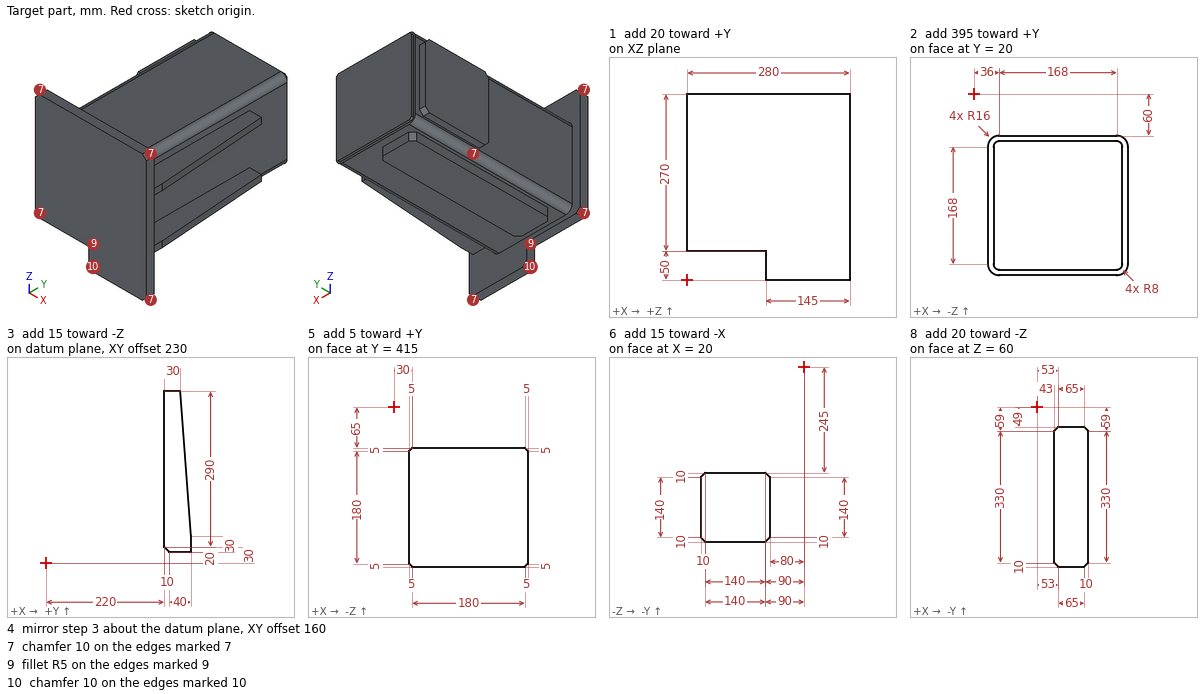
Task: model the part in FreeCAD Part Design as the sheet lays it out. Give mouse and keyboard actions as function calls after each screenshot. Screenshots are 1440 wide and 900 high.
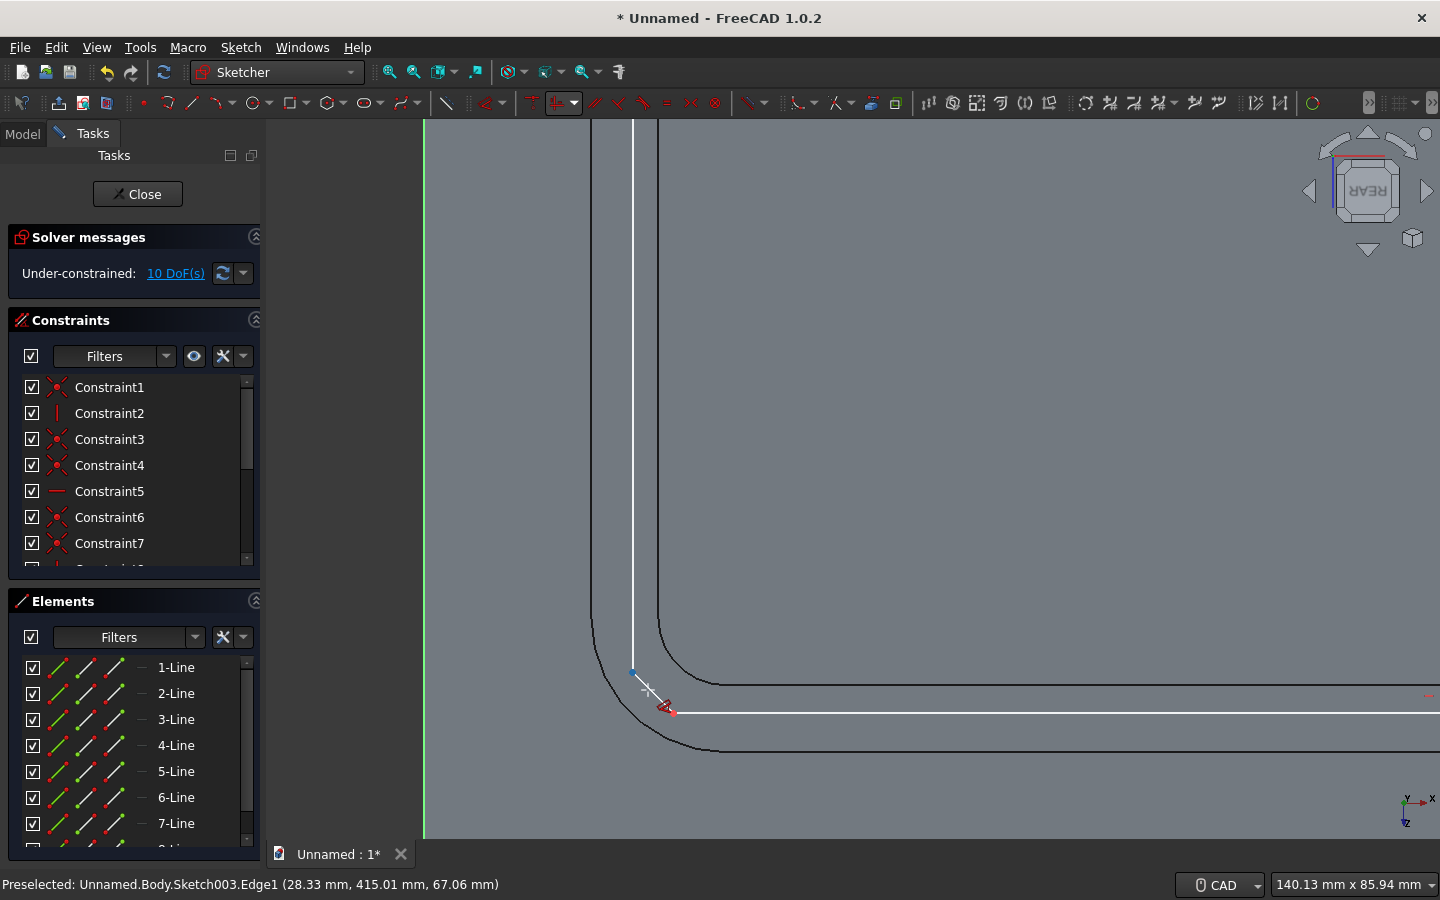
click(645, 685)
click(653, 747)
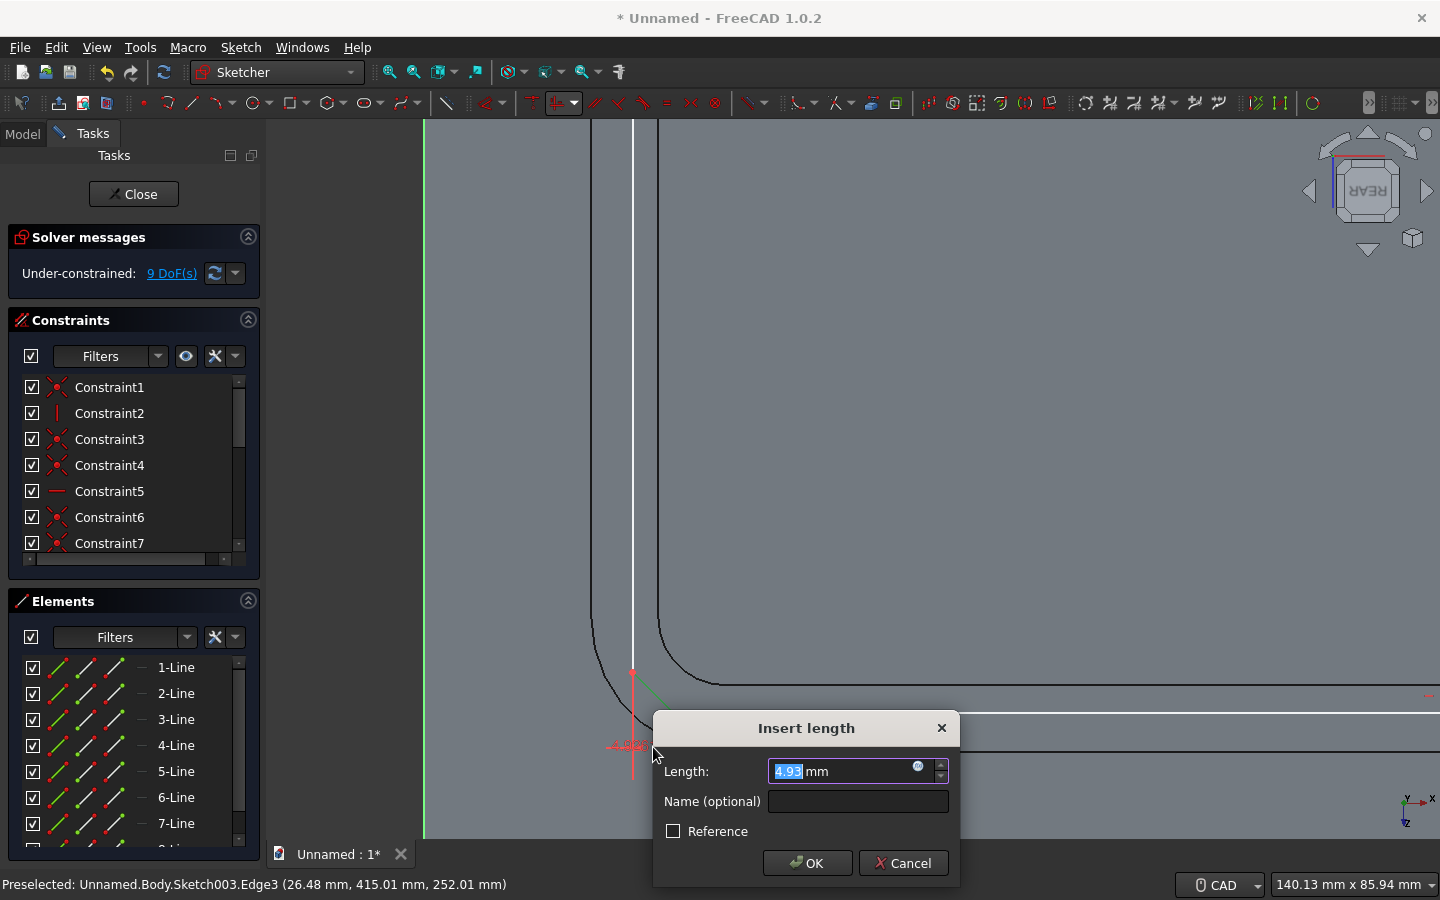
text(5)
key(Return)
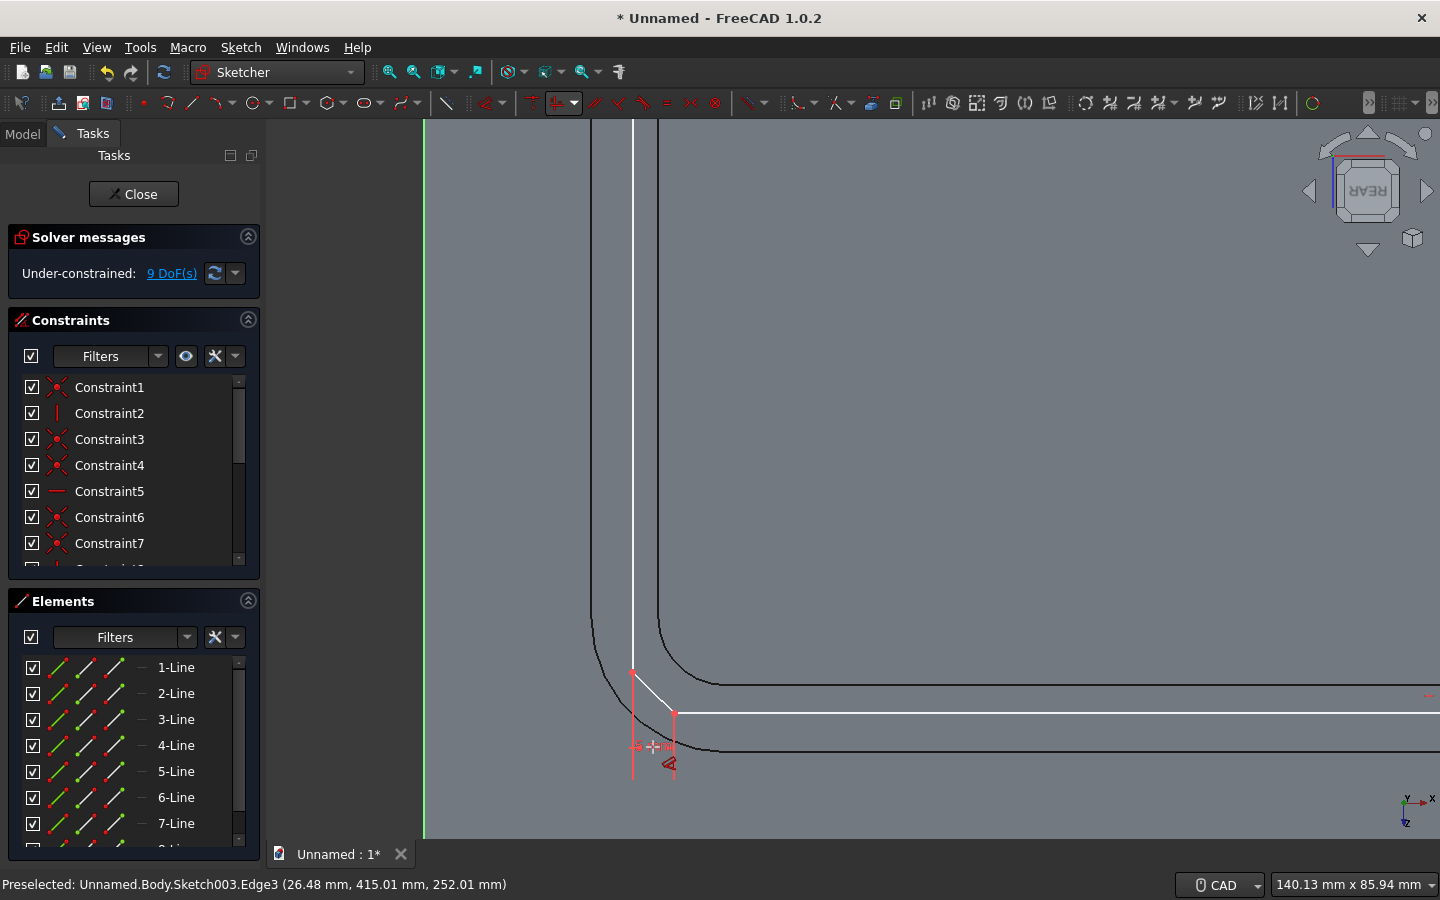
click(645, 685)
click(599, 693)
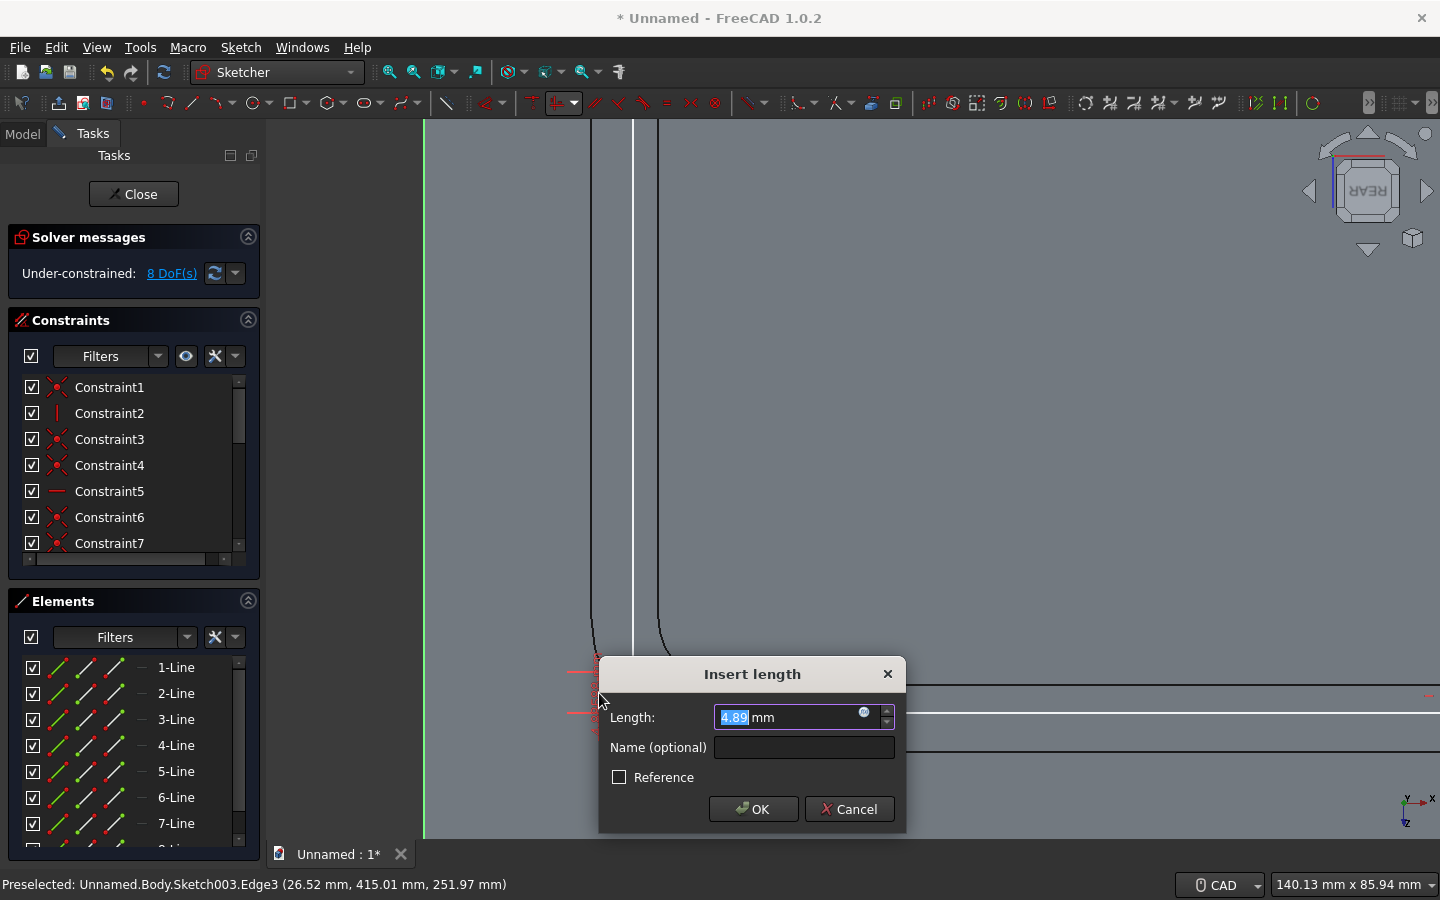
text(5)
key(Return)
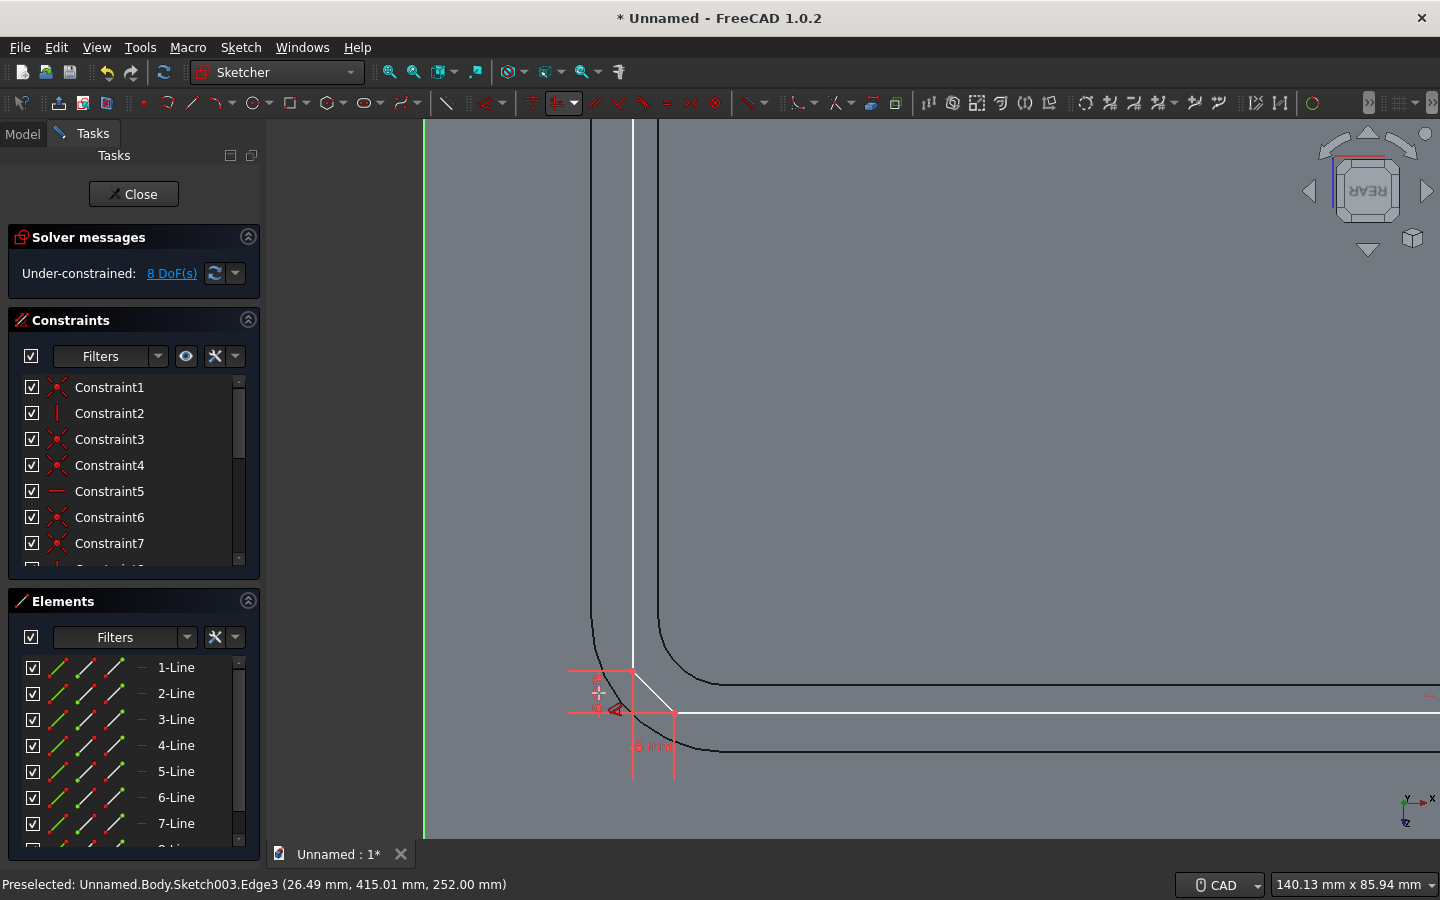
scroll(648, 691, down, 8)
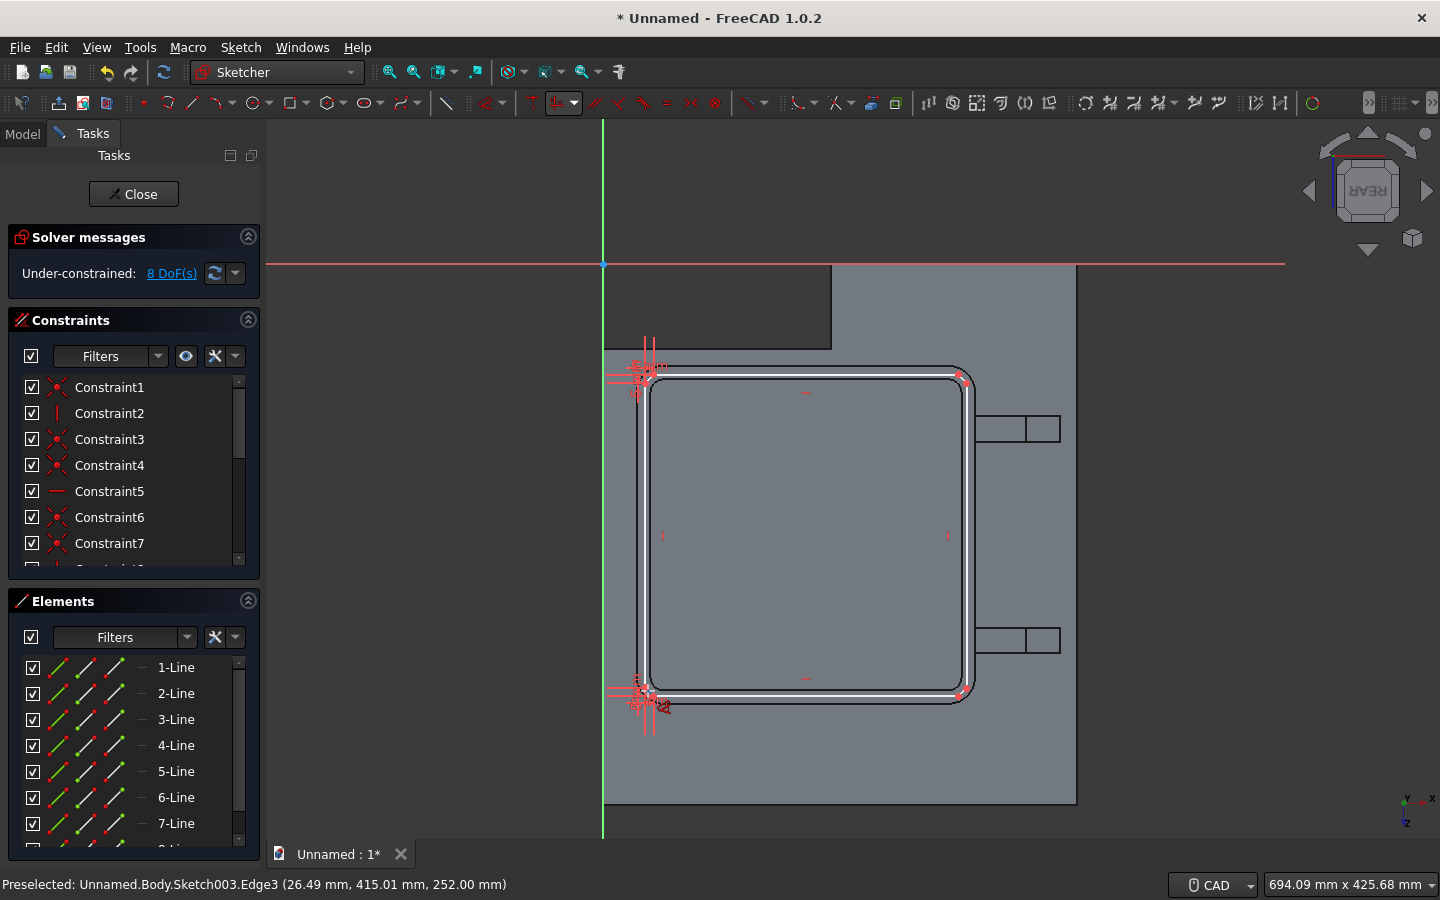
scroll(961, 694, up, 8)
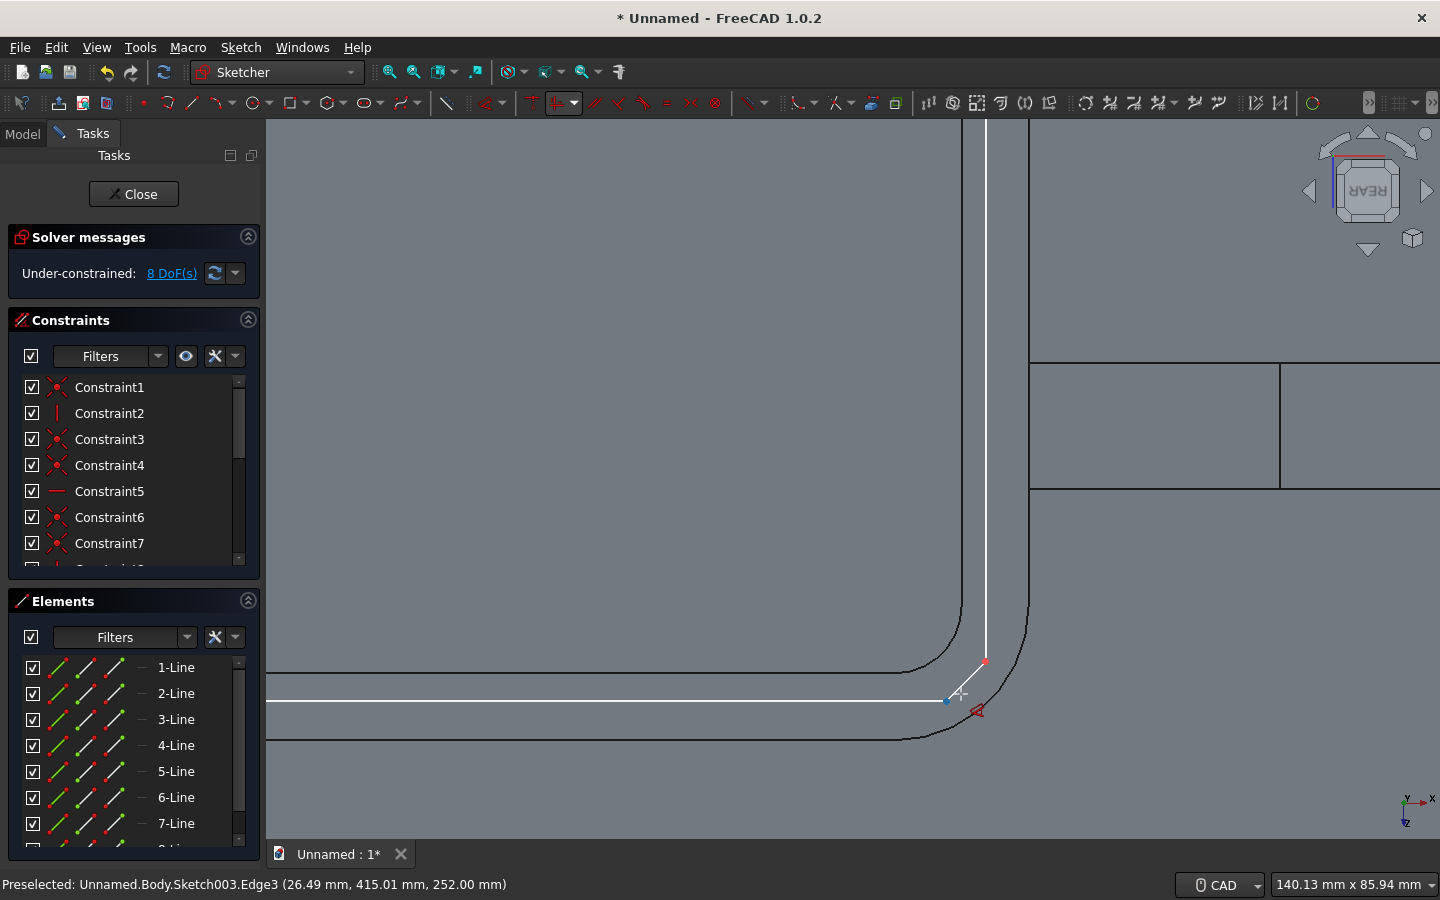
click(958, 689)
click(966, 735)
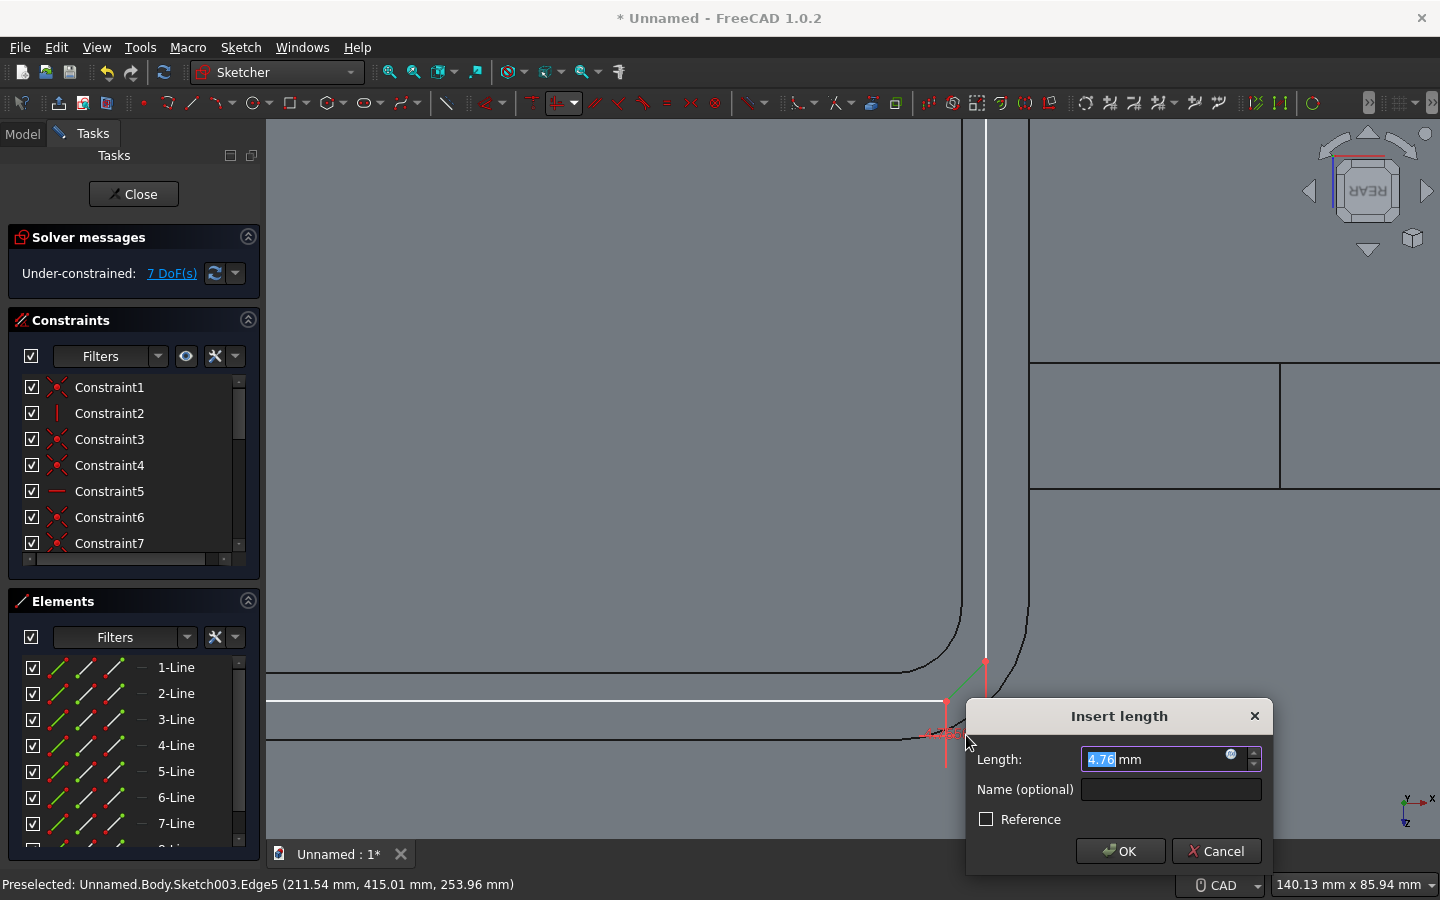
text(5)
key(Return)